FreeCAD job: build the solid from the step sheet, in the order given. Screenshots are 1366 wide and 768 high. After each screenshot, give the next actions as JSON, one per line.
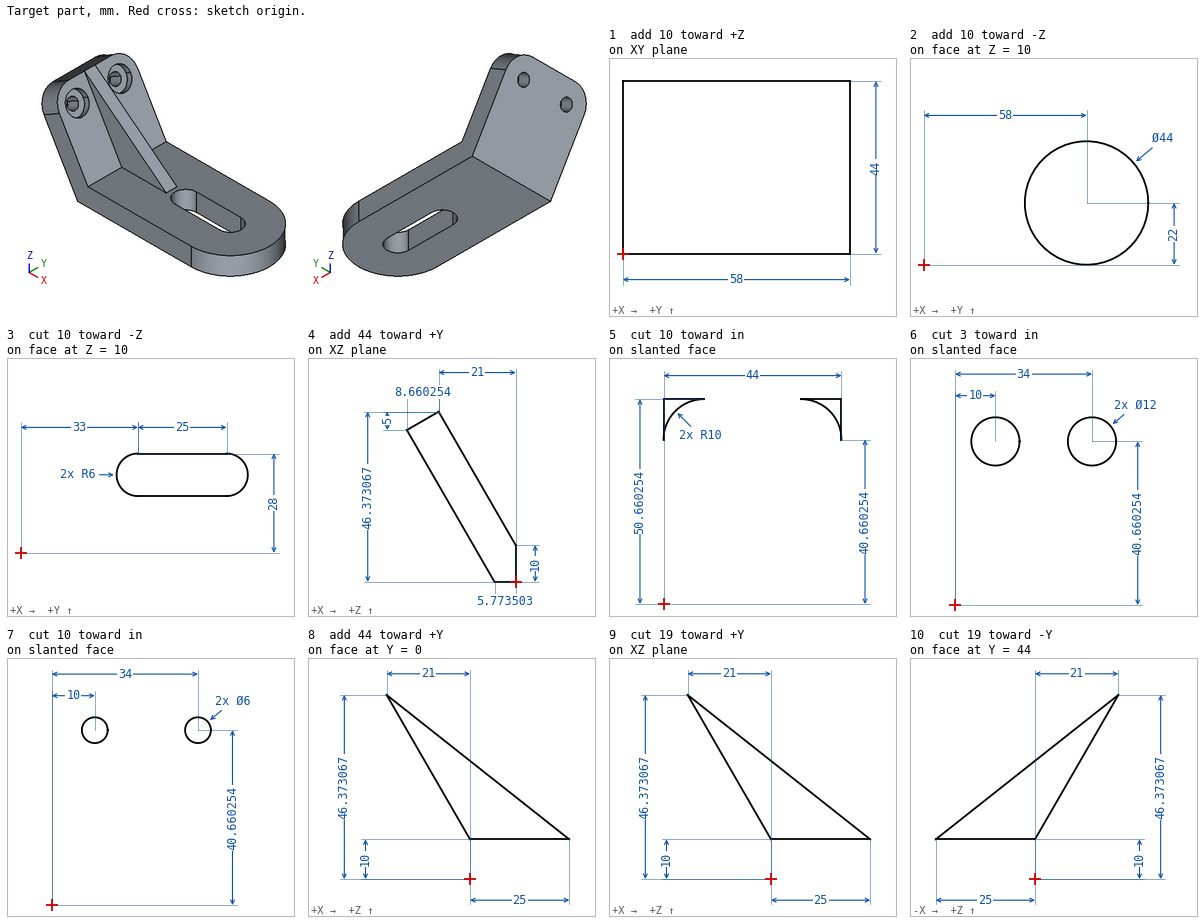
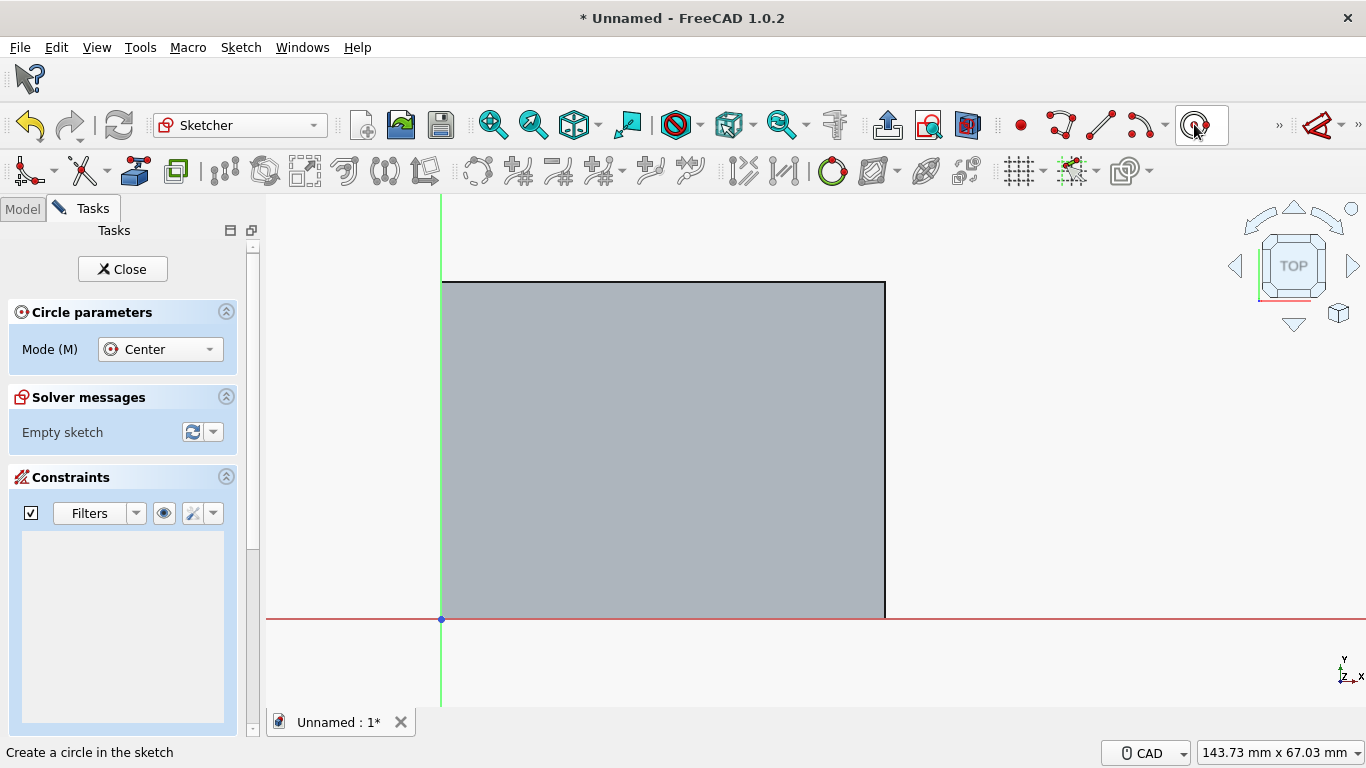
{"action": "left_click", "coordinate": [885, 451]}
{"action": "mouse_move", "coordinate": [1004, 332]}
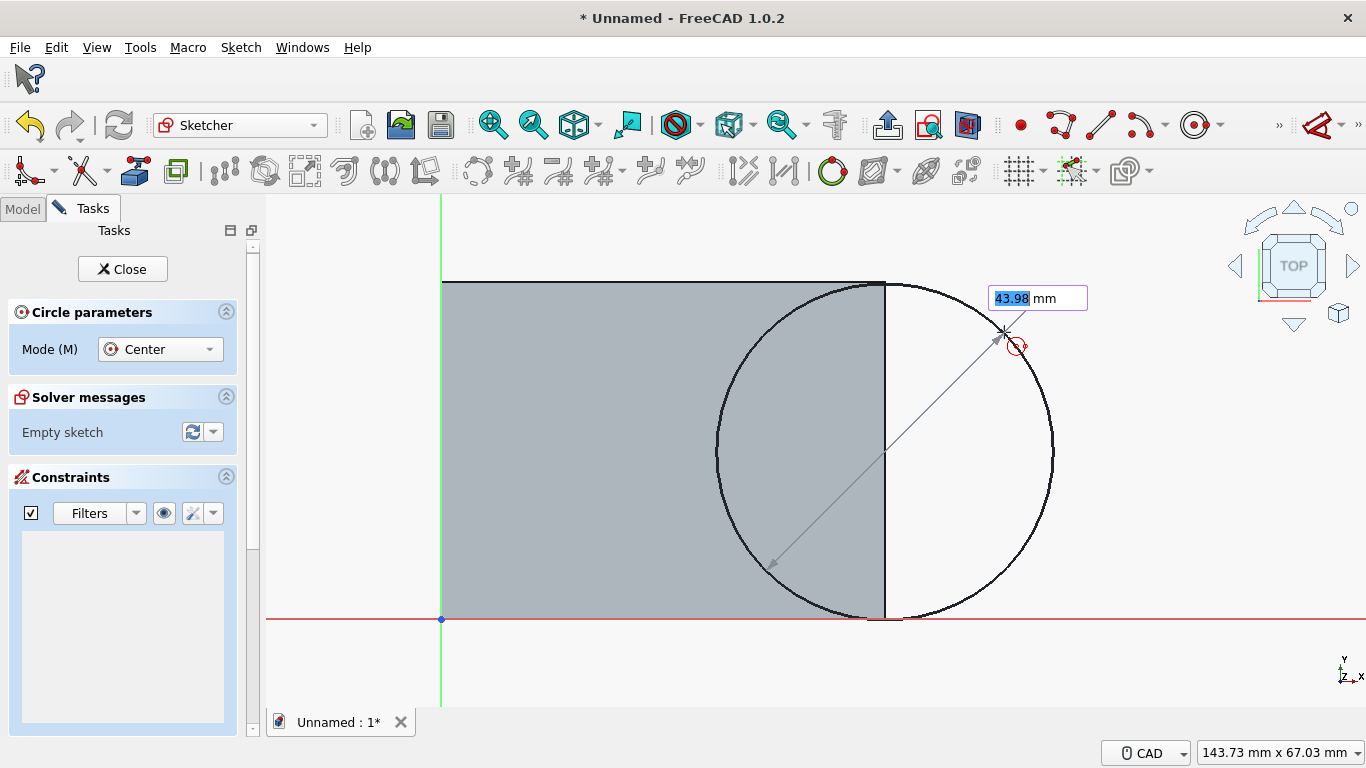
{"action": "type", "text": "44"}
{"action": "key", "text": "Return"}
{"action": "key", "text": "Escape"}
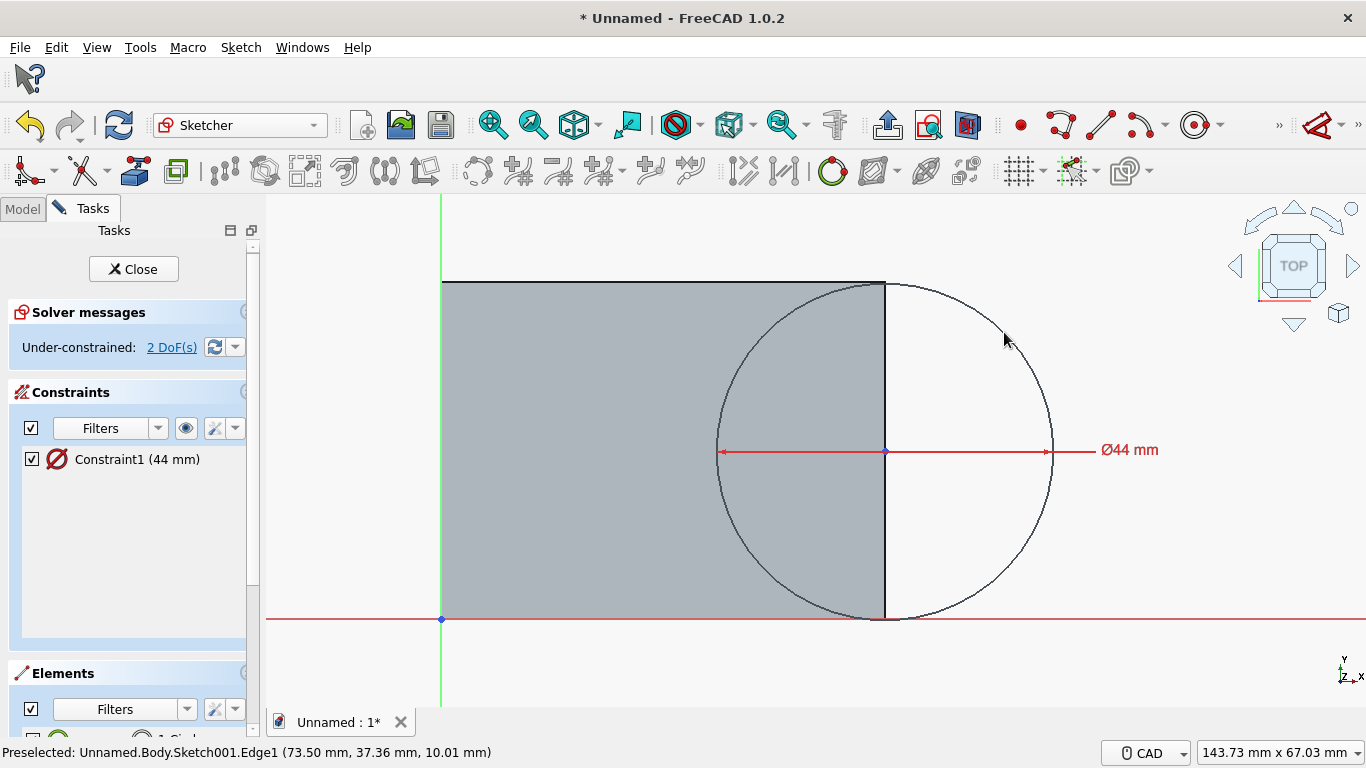
{"action": "left_click", "coordinate": [1318, 126]}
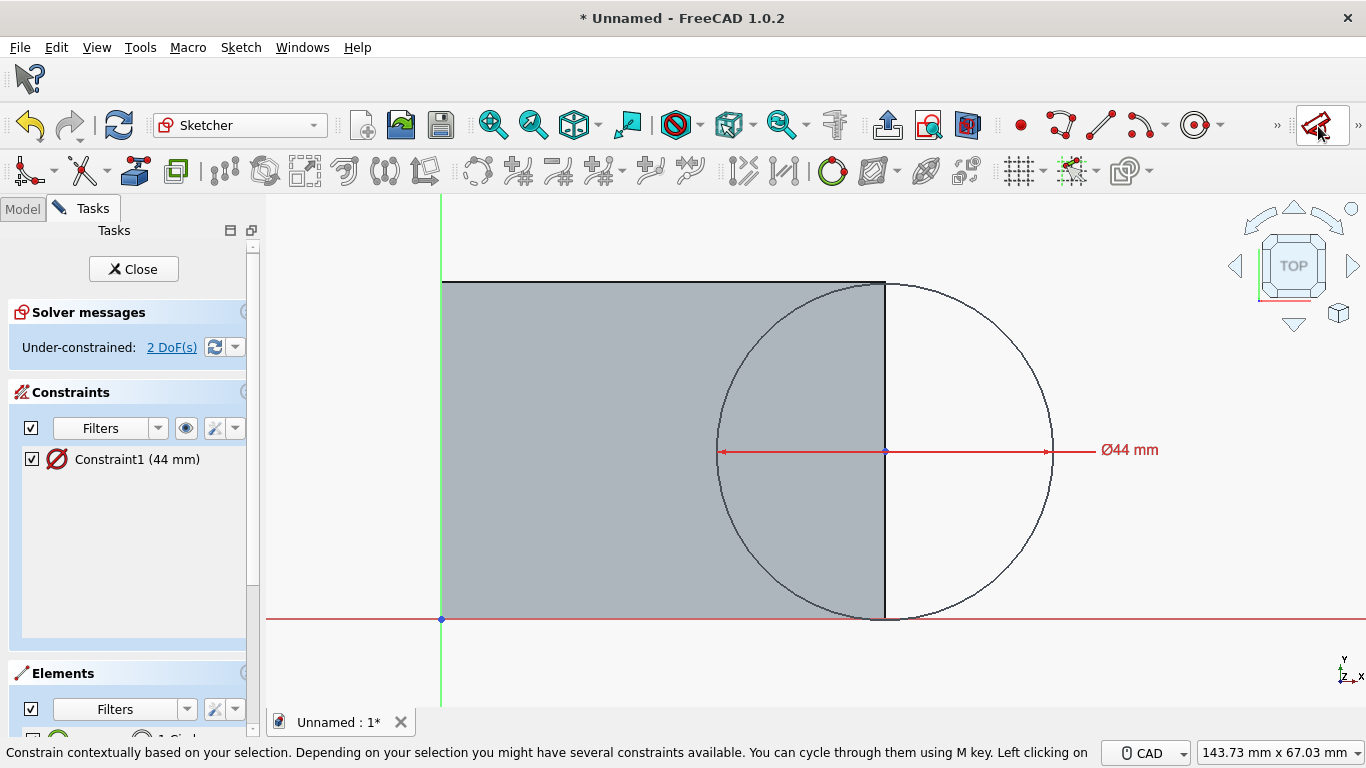
{"action": "left_click", "coordinate": [885, 452]}
{"action": "left_click", "coordinate": [663, 653]}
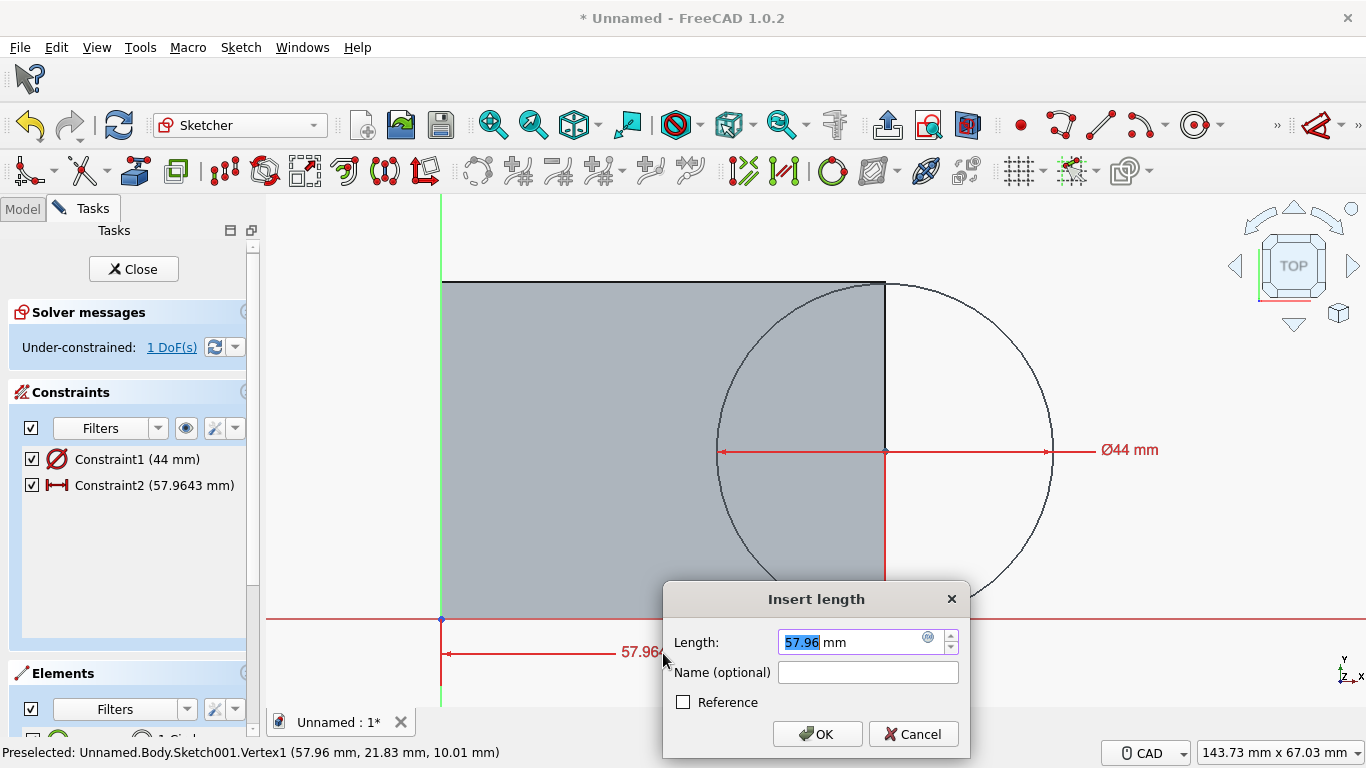
{"action": "type", "text": "58"}
{"action": "key", "text": "Return"}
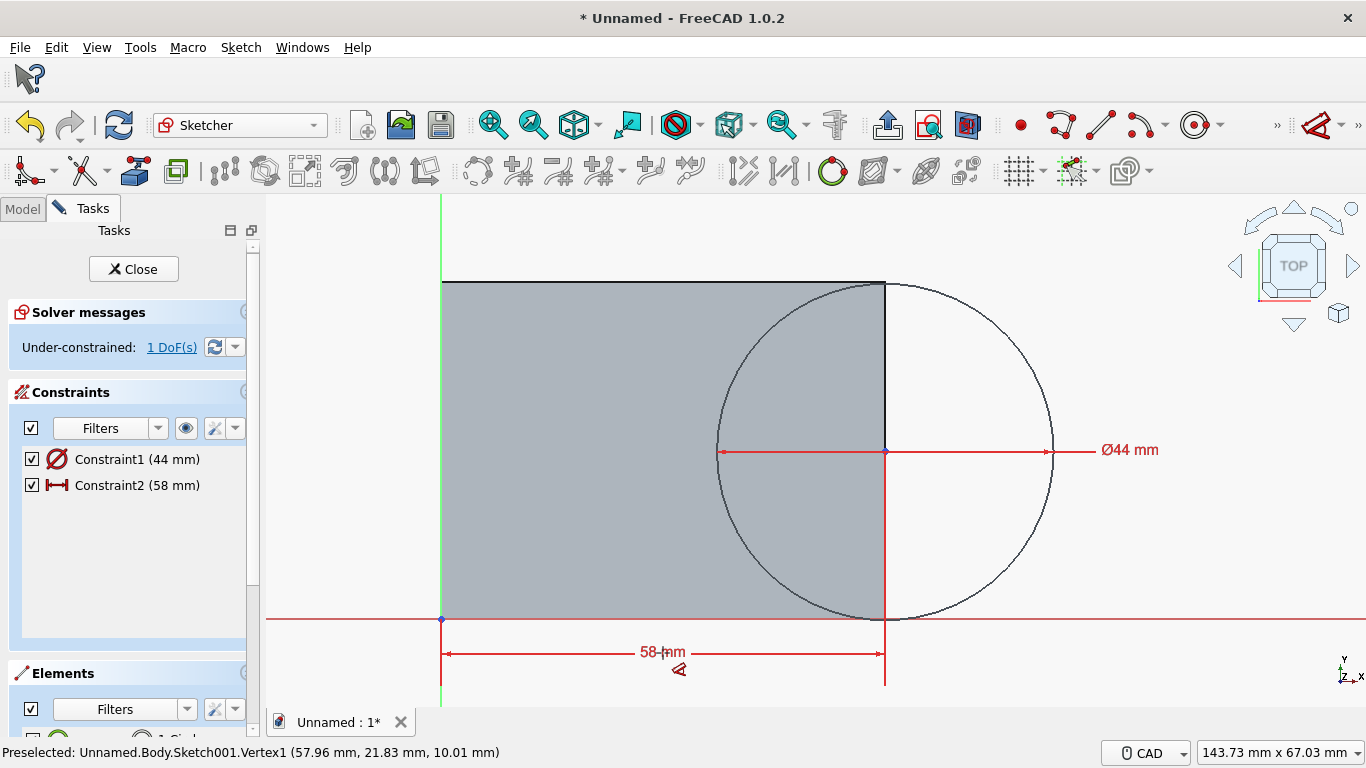
{"action": "left_click", "coordinate": [885, 452]}
{"action": "left_click", "coordinate": [407, 536]}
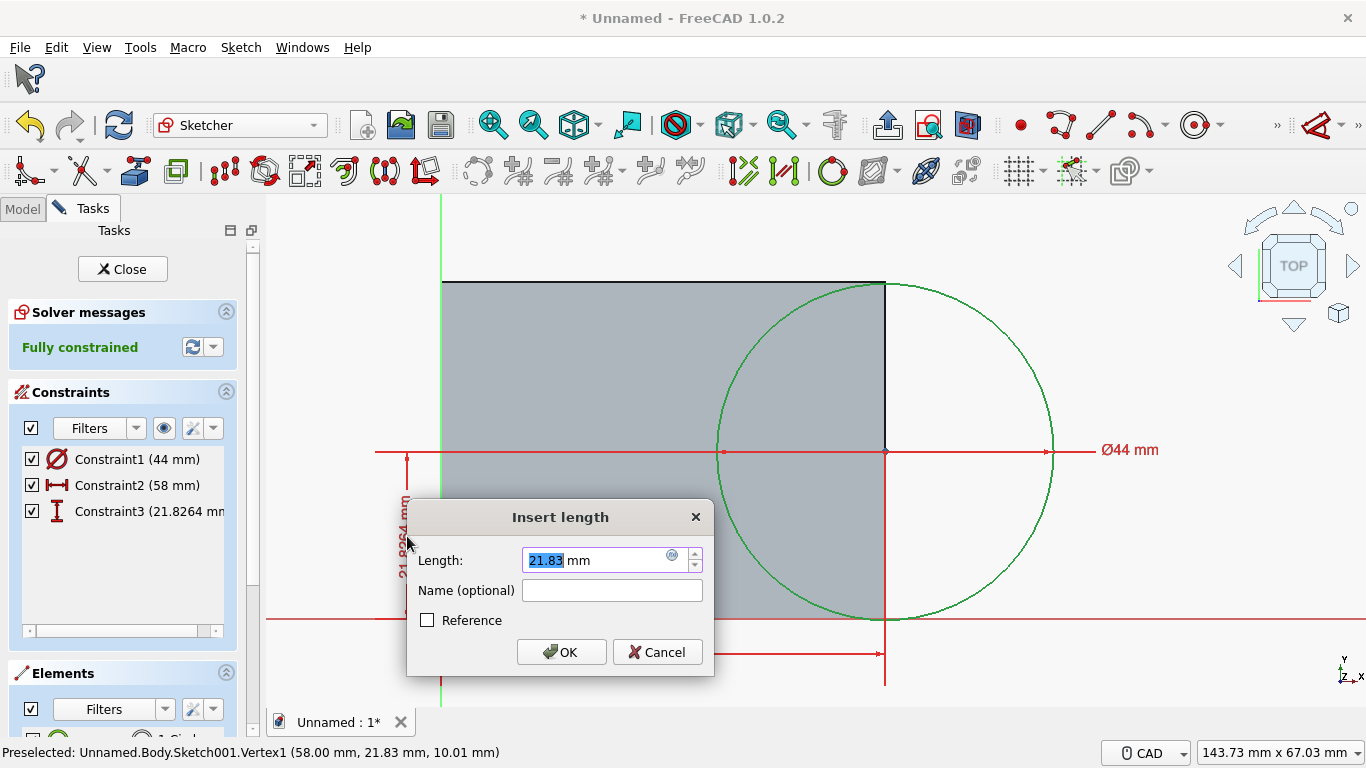
{"action": "type", "text": "22"}
{"action": "key", "text": "Return"}
{"action": "key", "text": "Escape"}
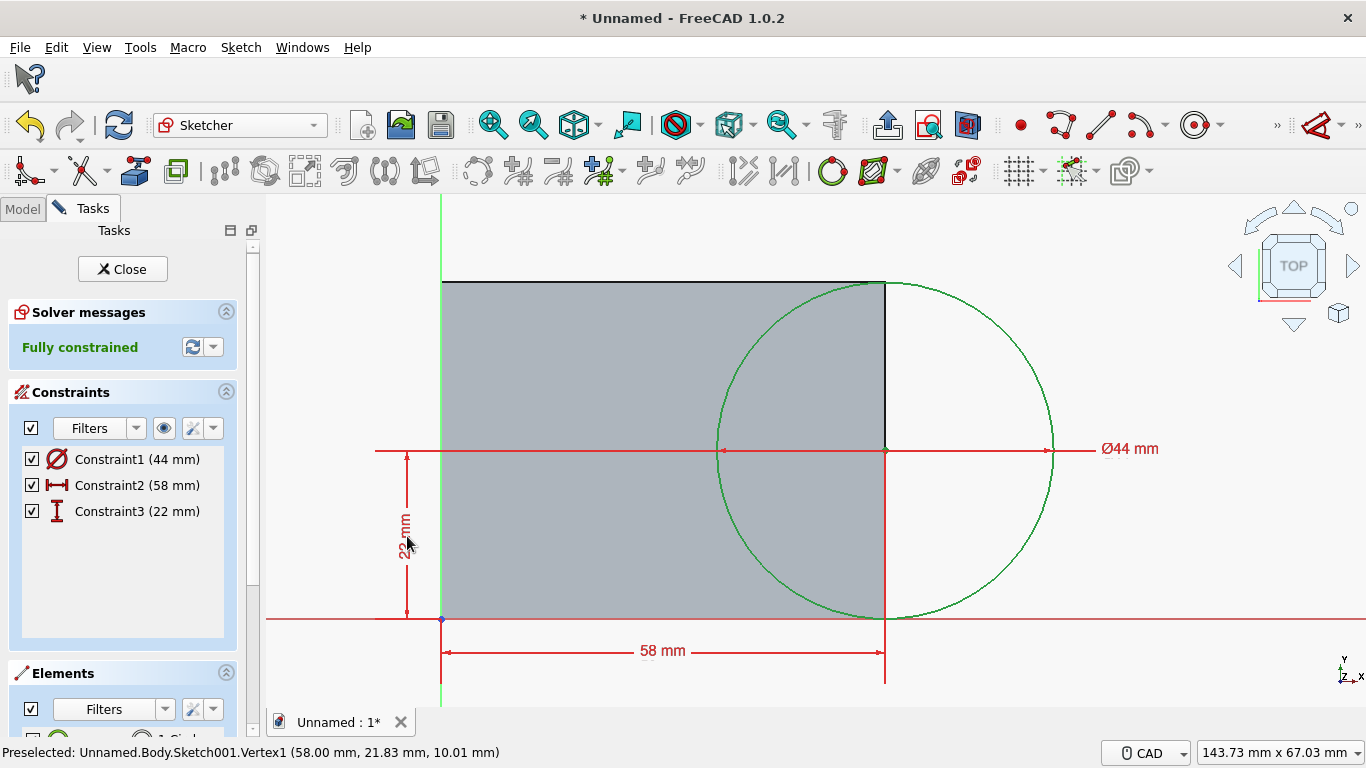
{"action": "left_click", "coordinate": [123, 269]}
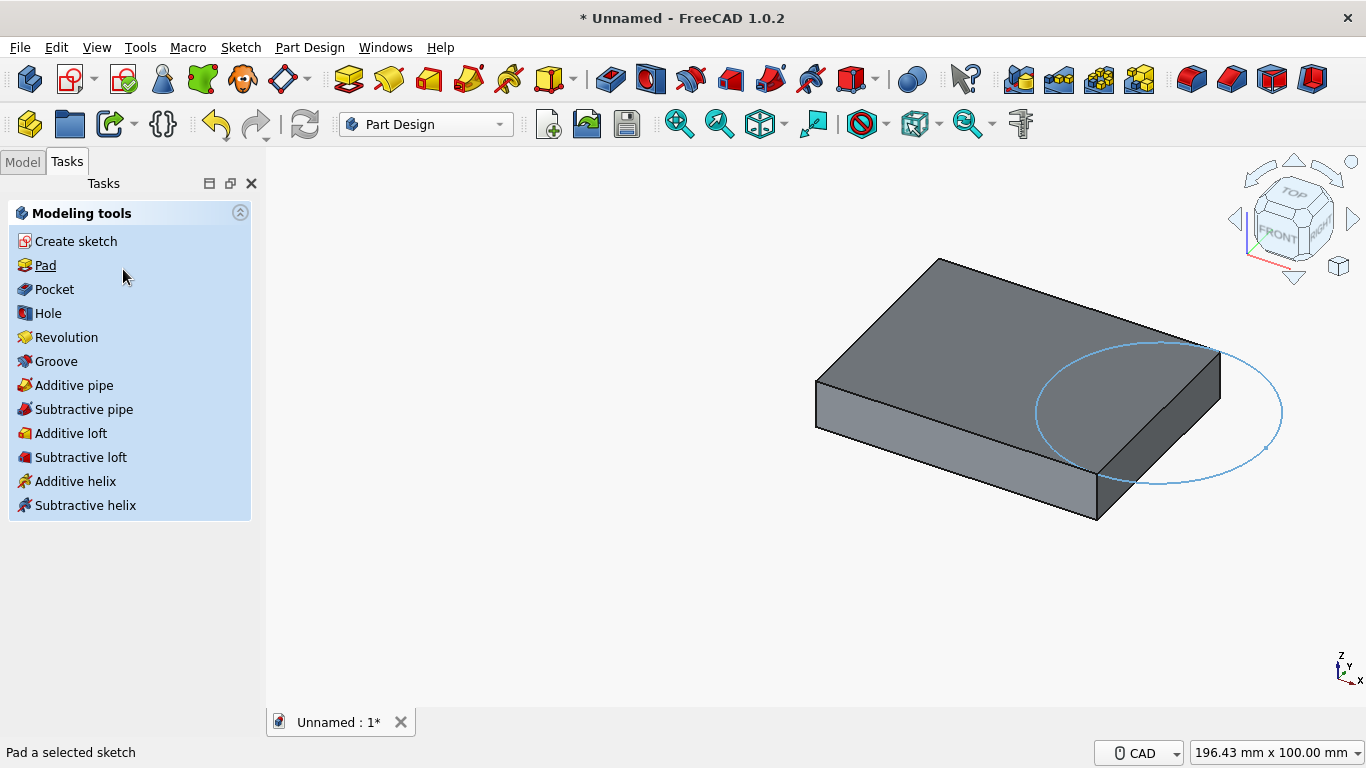
{"action": "left_click", "coordinate": [350, 80]}